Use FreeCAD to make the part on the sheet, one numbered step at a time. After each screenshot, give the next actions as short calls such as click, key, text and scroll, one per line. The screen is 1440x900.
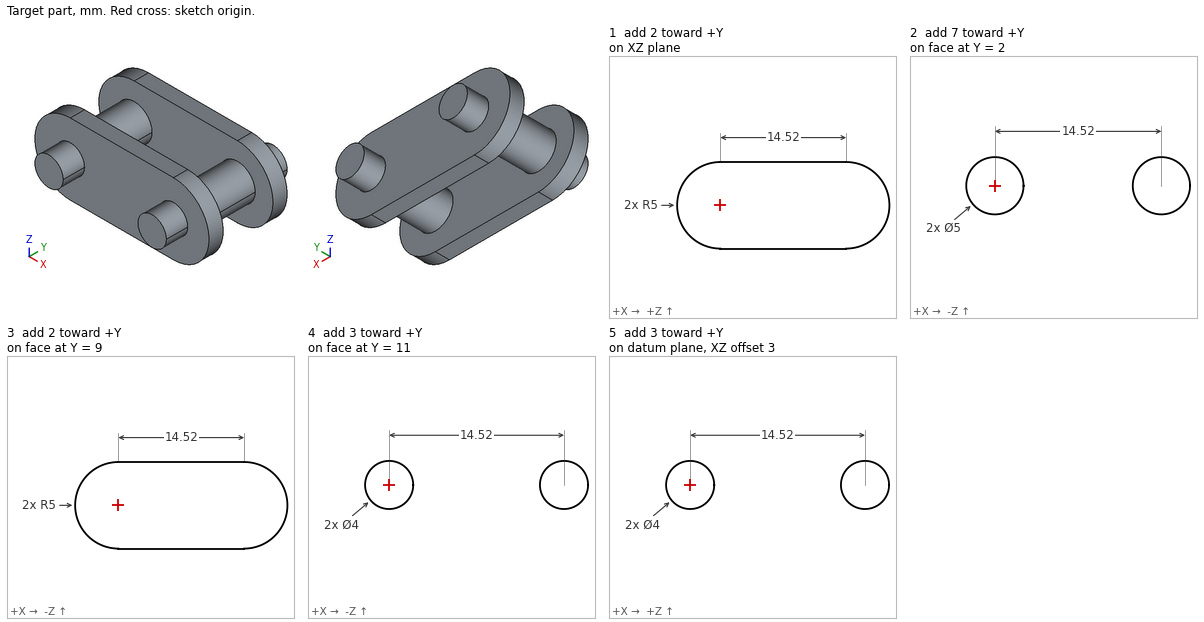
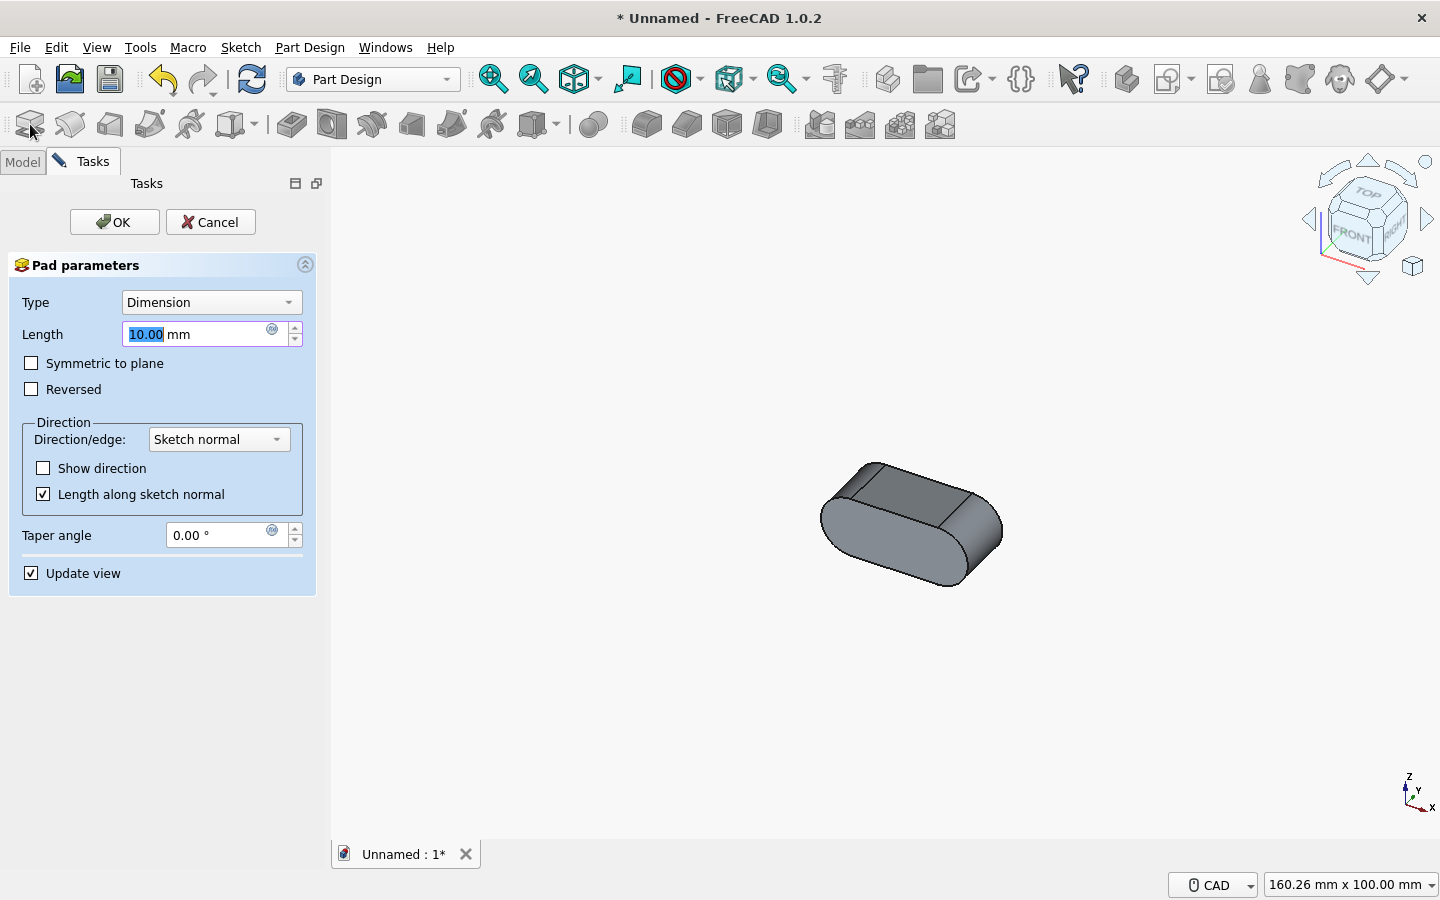
text(2)
key(Tab)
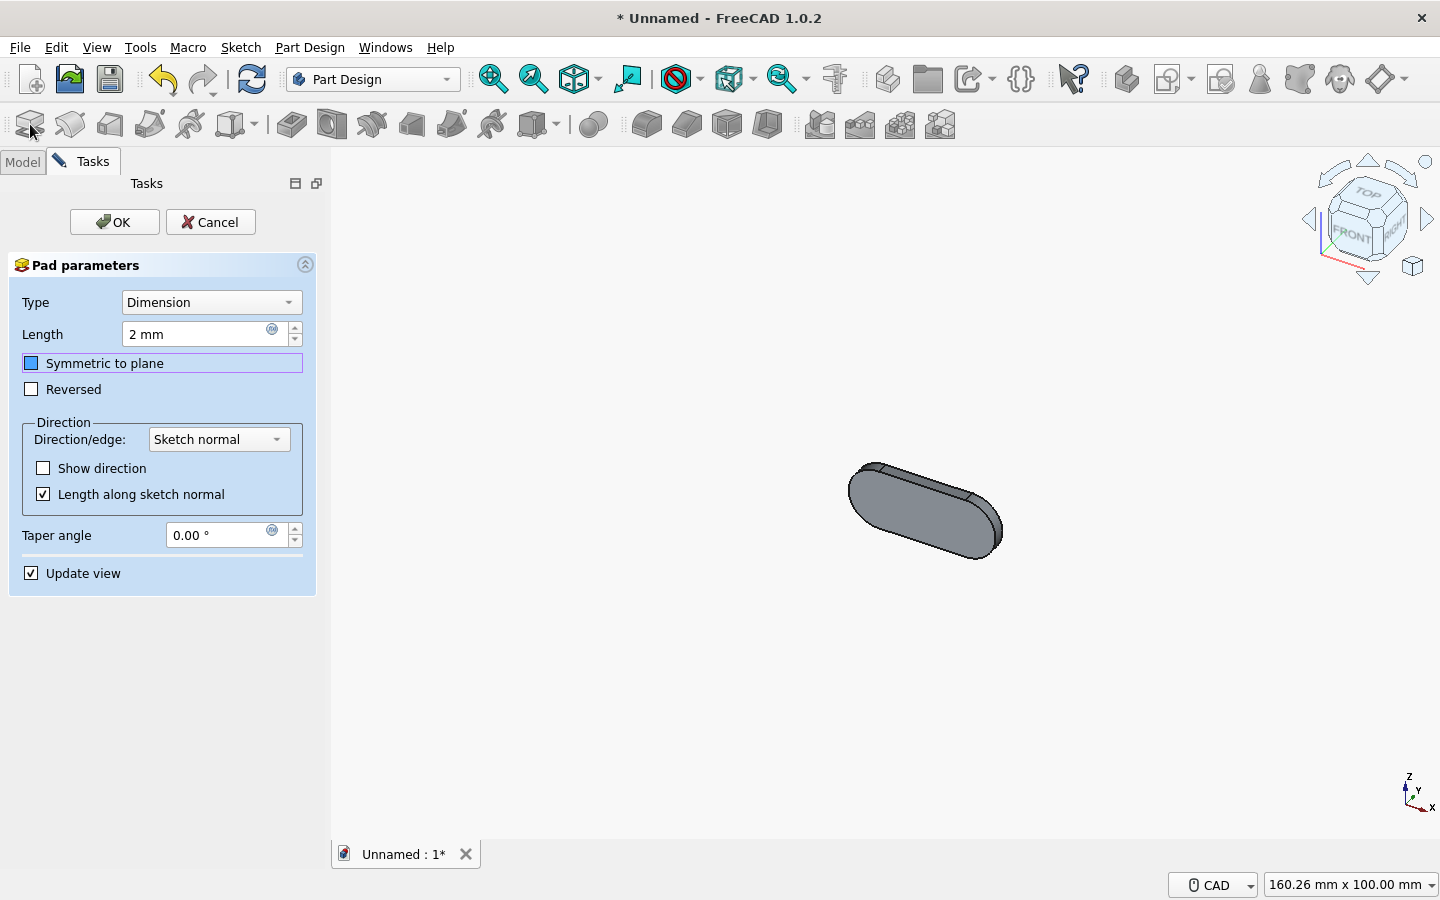
click(30, 389)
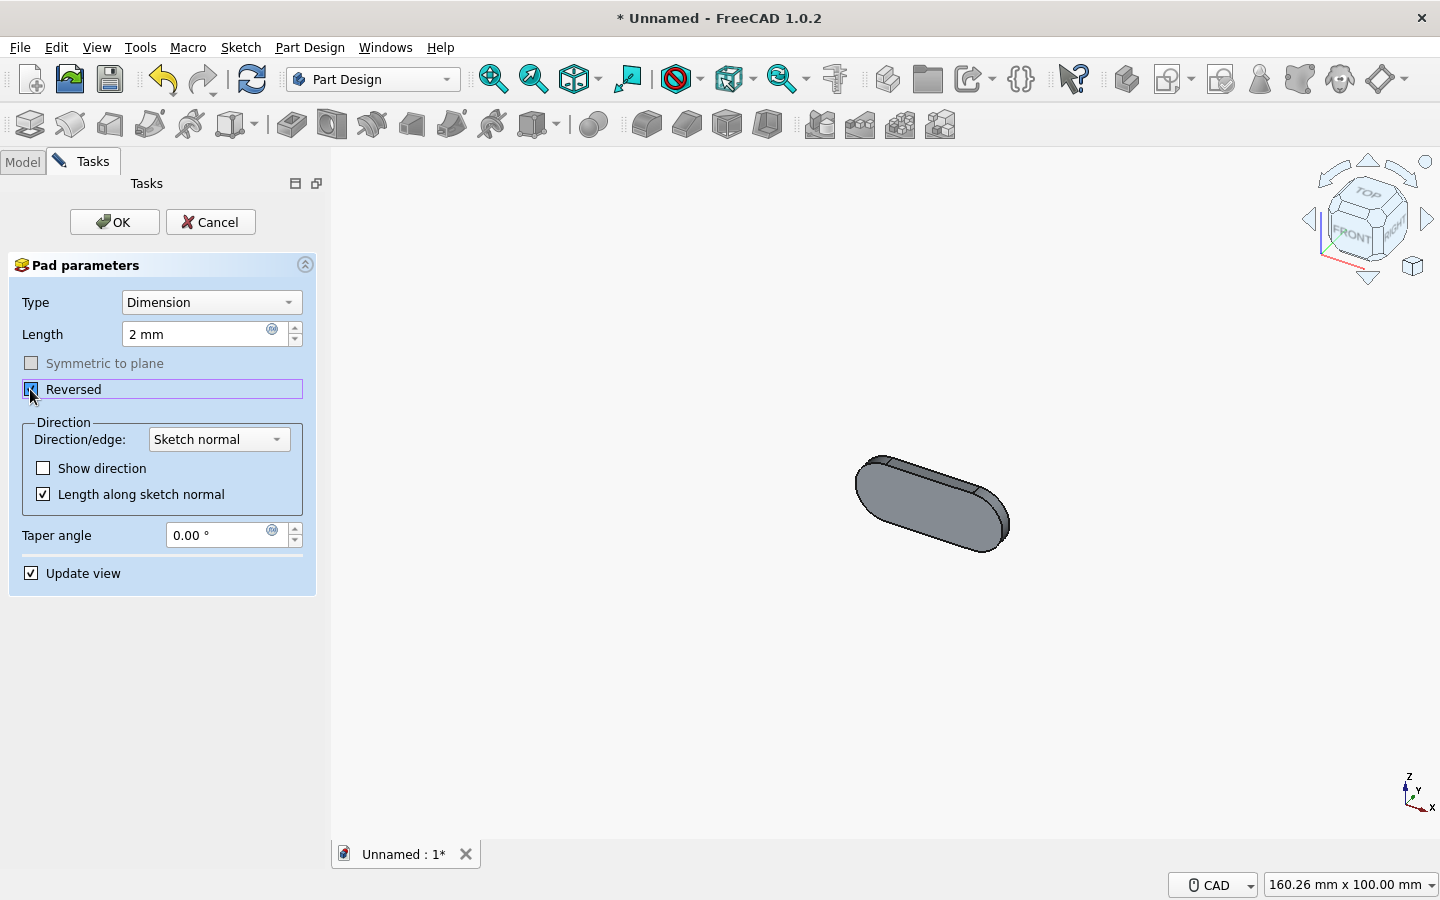
click(115, 222)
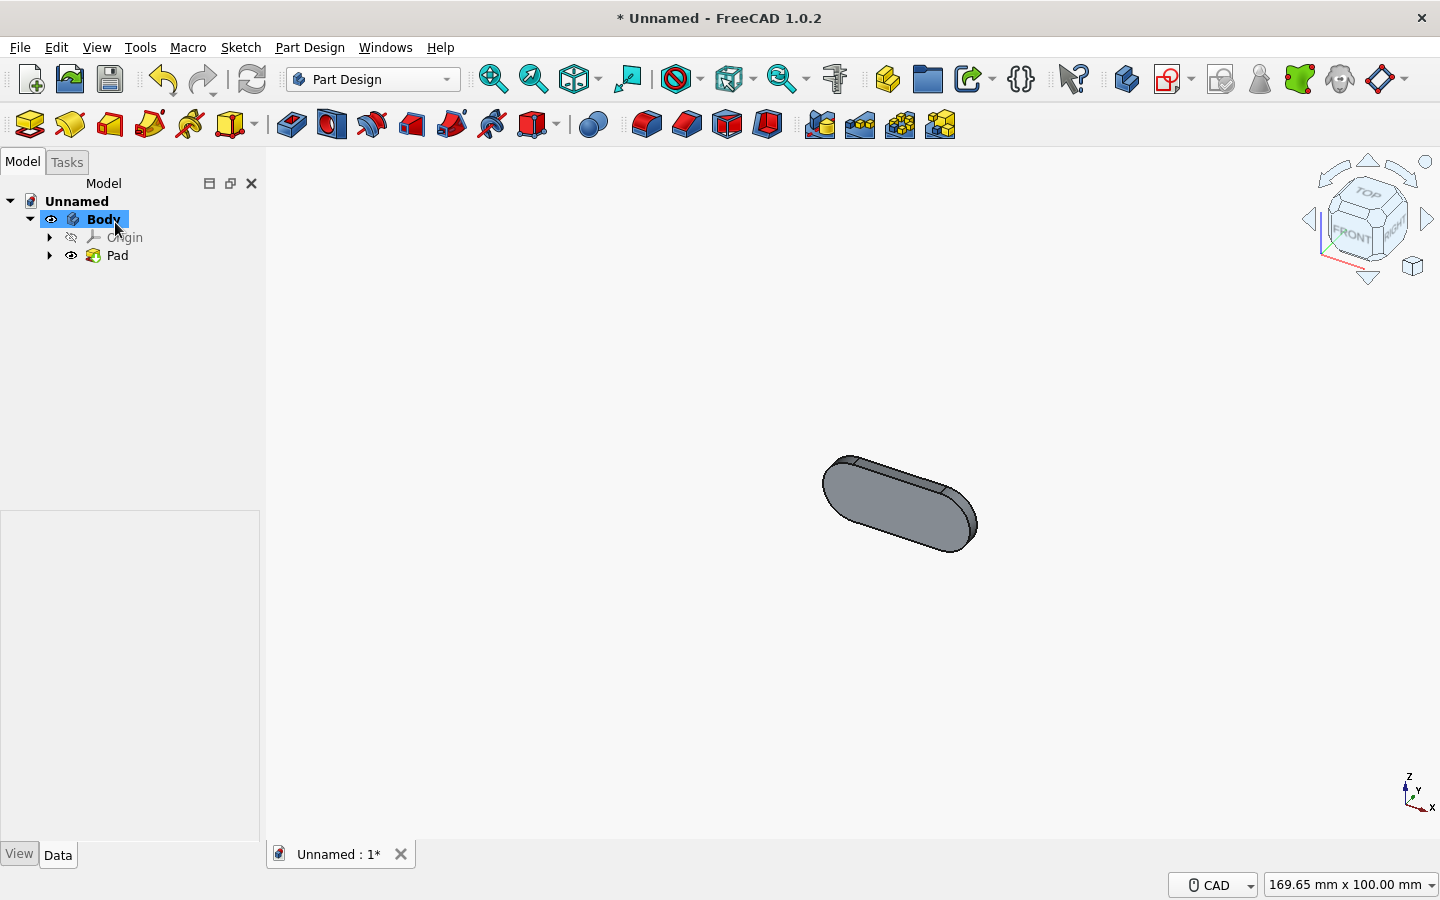
click(494, 80)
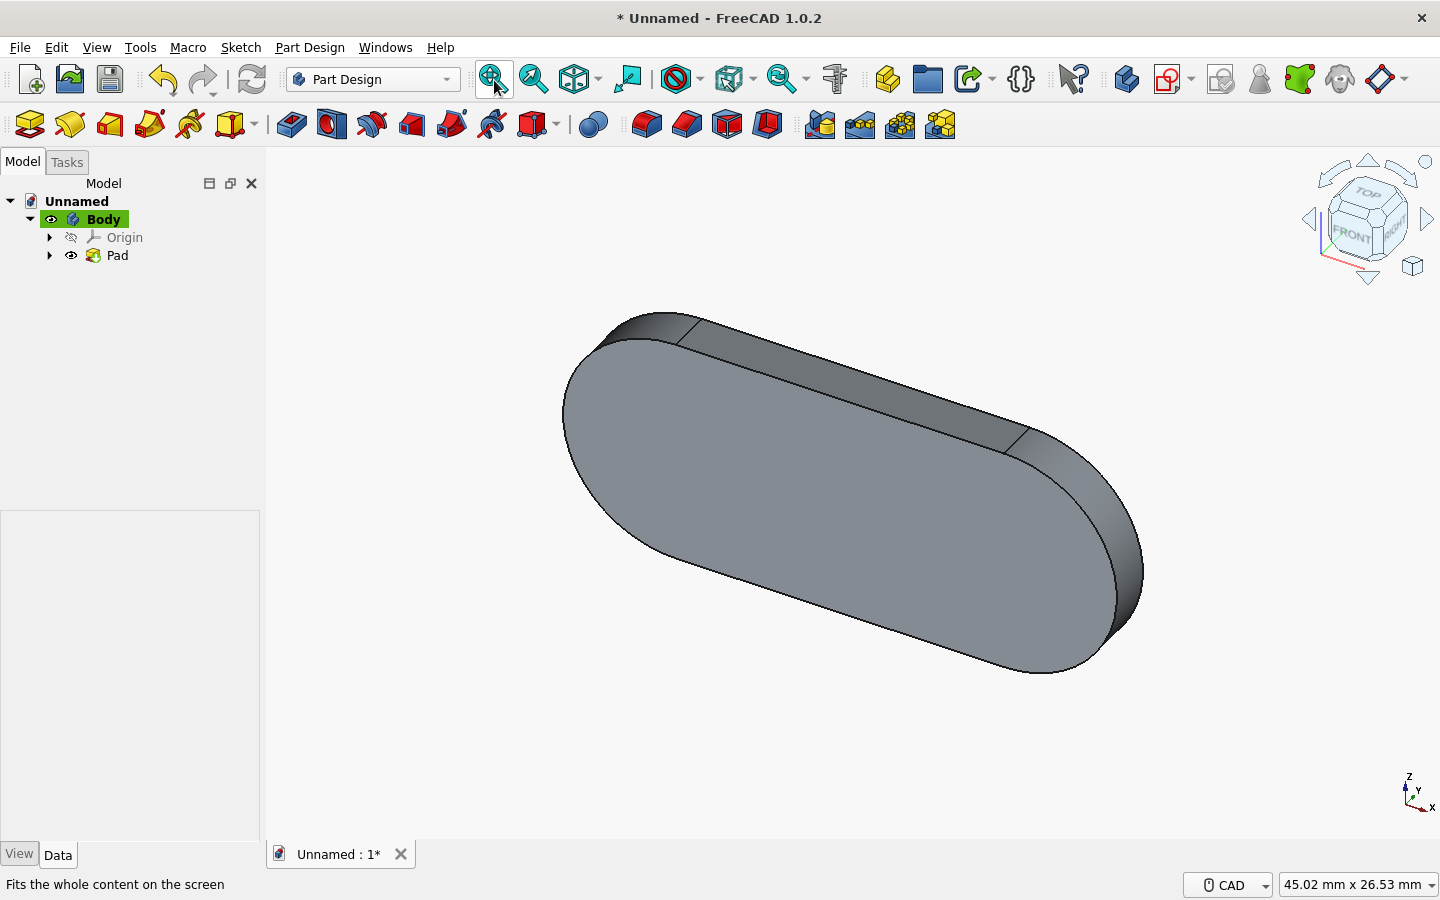
key(4)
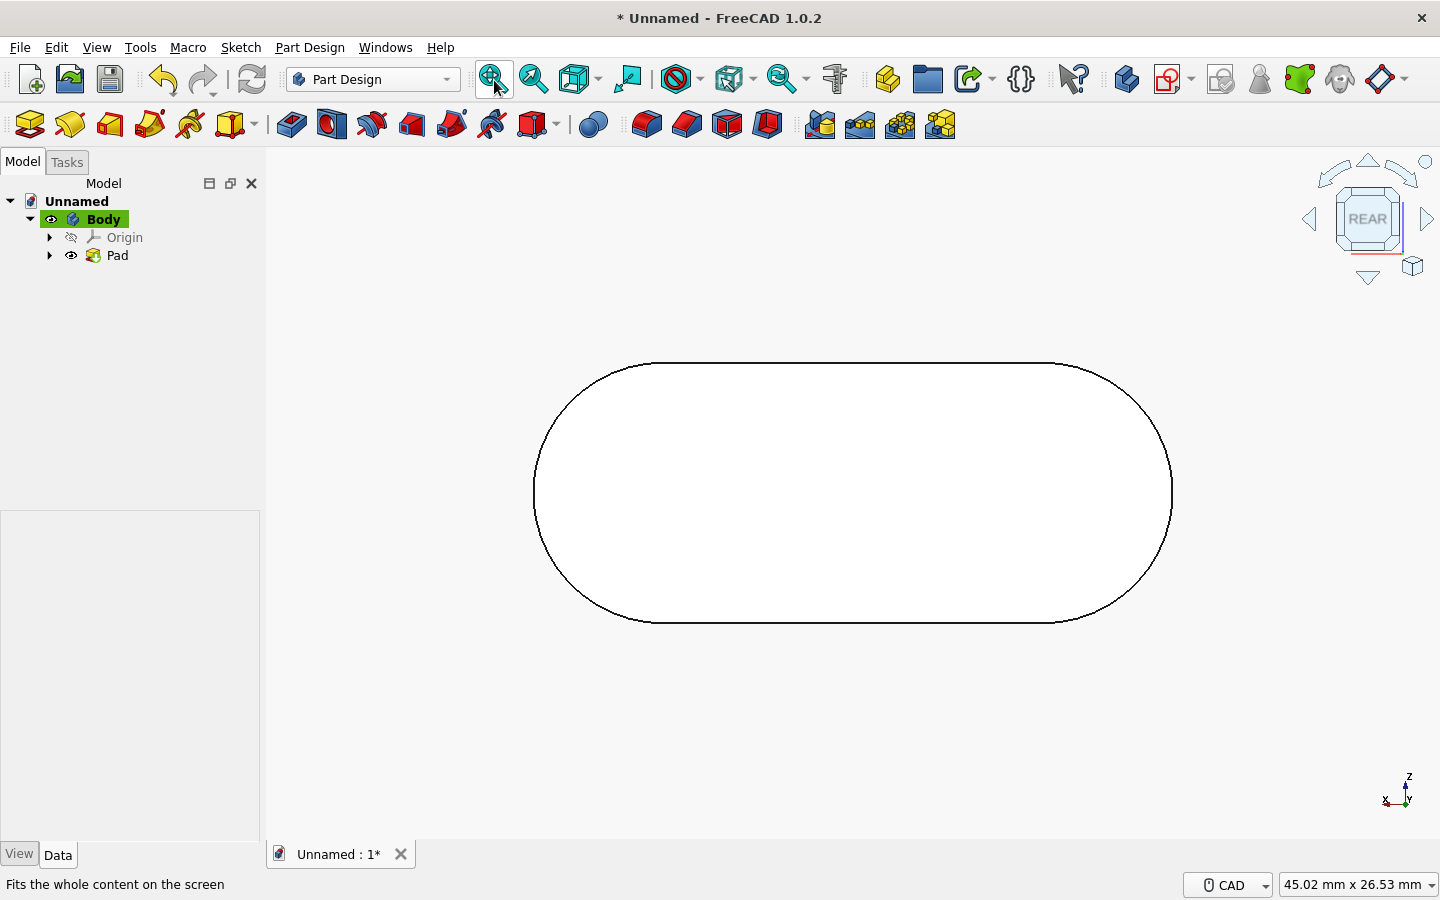
click(670, 492)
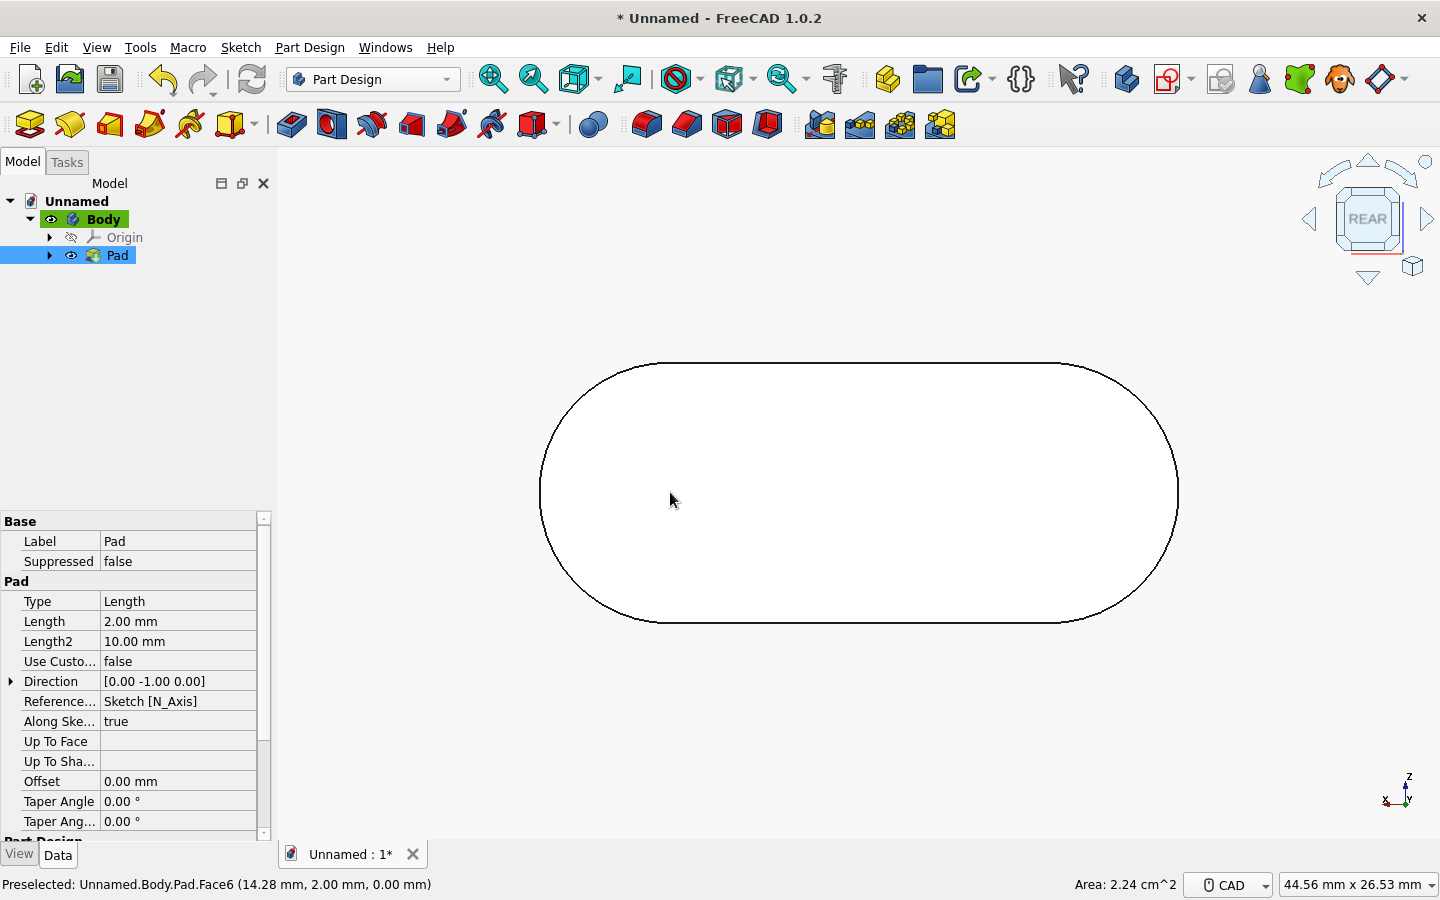
click(1168, 80)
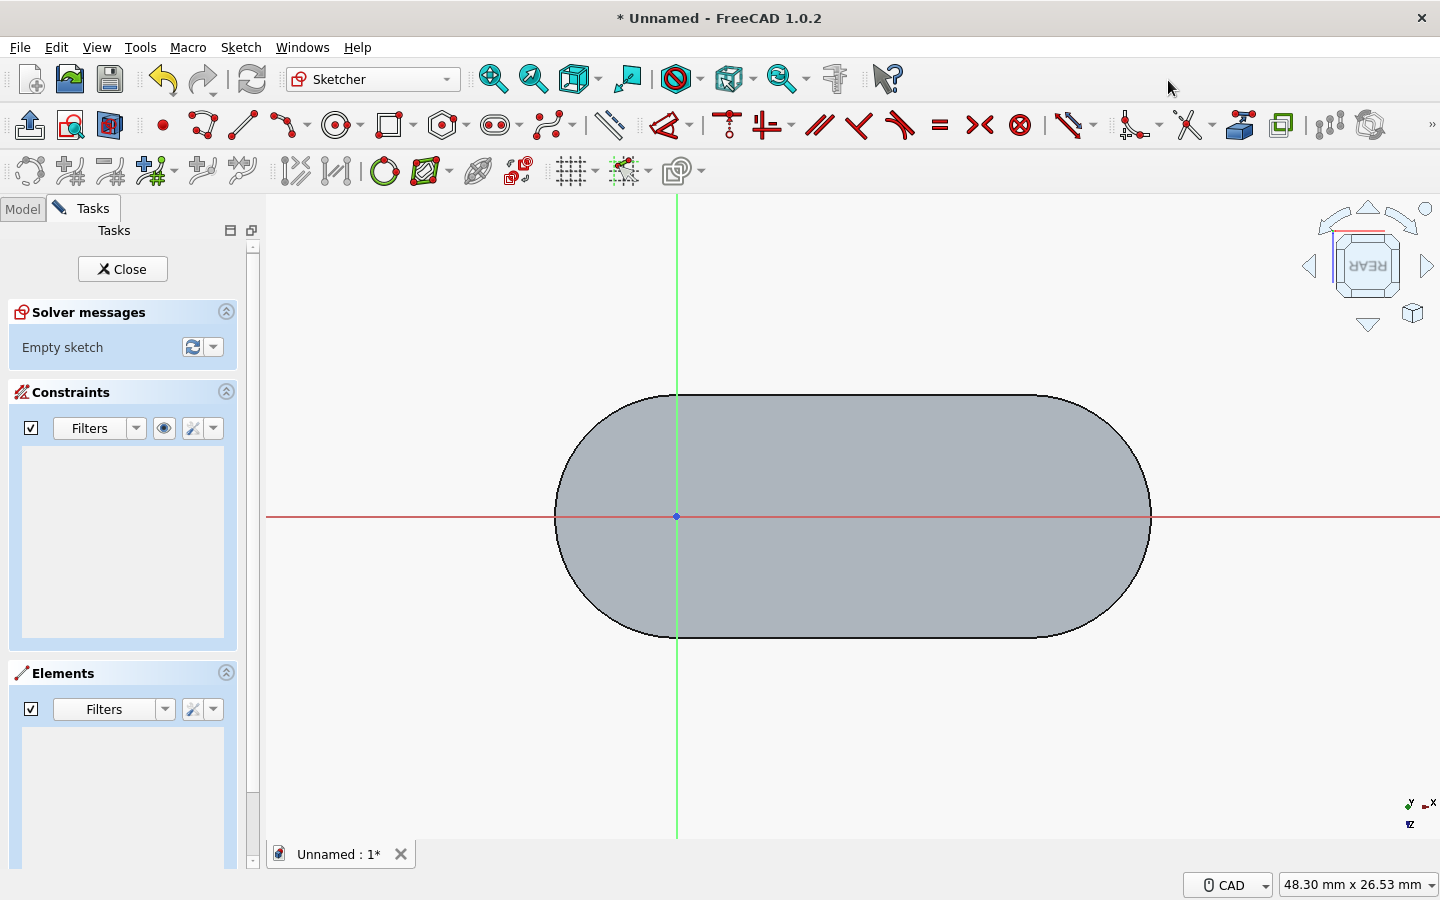
scroll(992, 517, up, 2)